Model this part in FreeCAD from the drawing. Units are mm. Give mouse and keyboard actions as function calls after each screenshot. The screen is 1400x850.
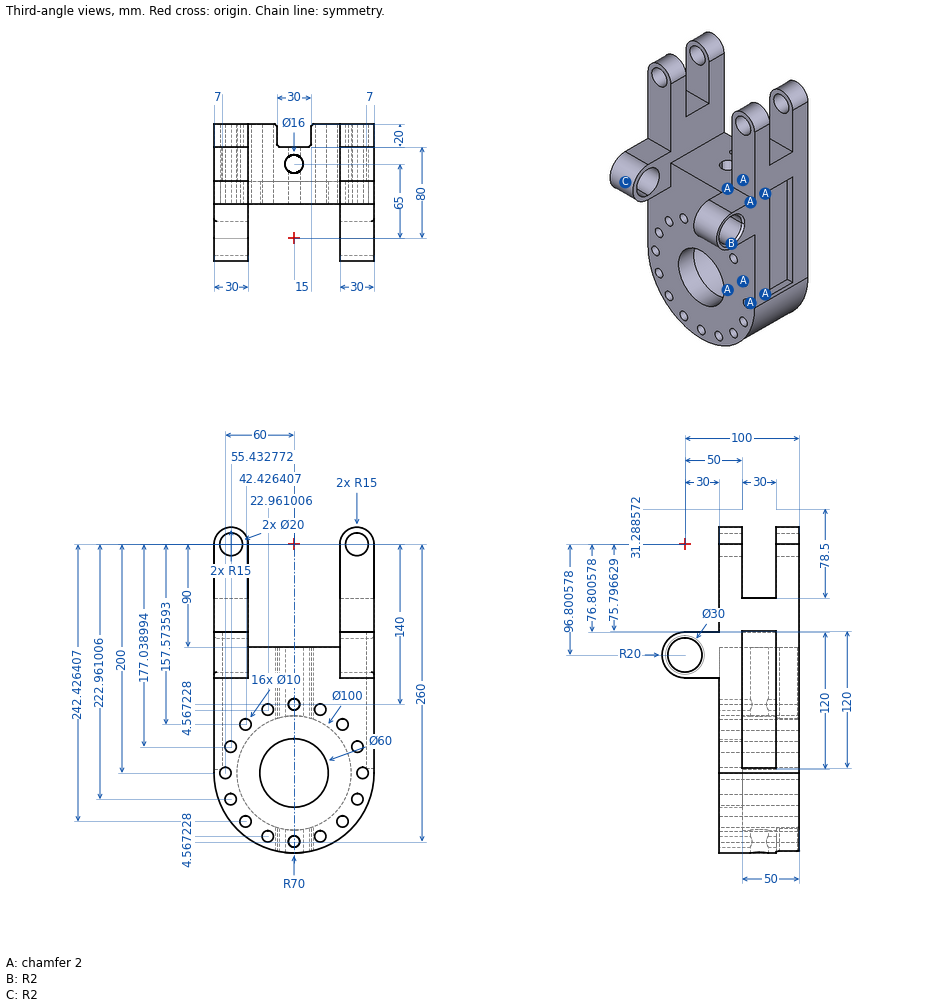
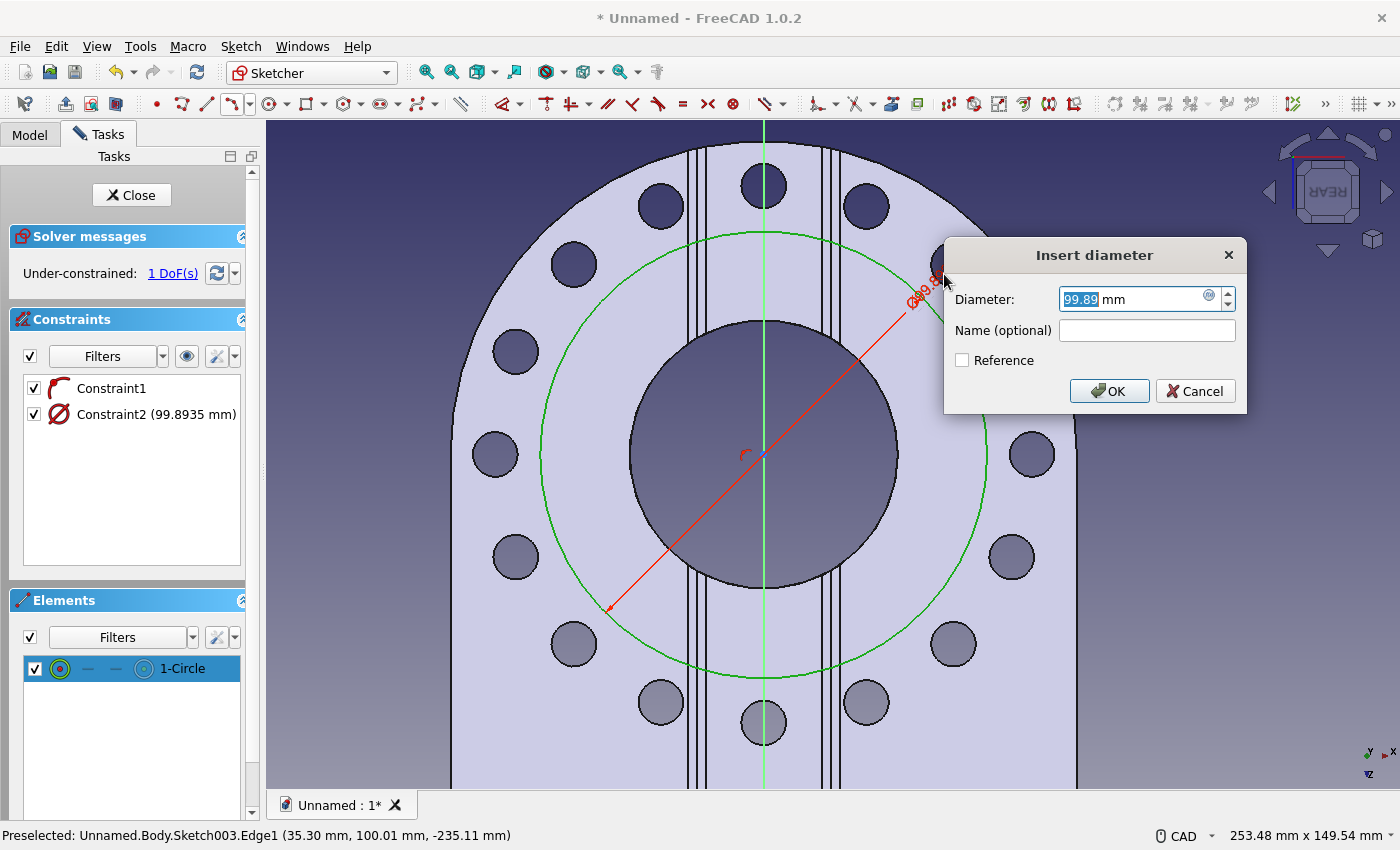
text(100)
key(Return)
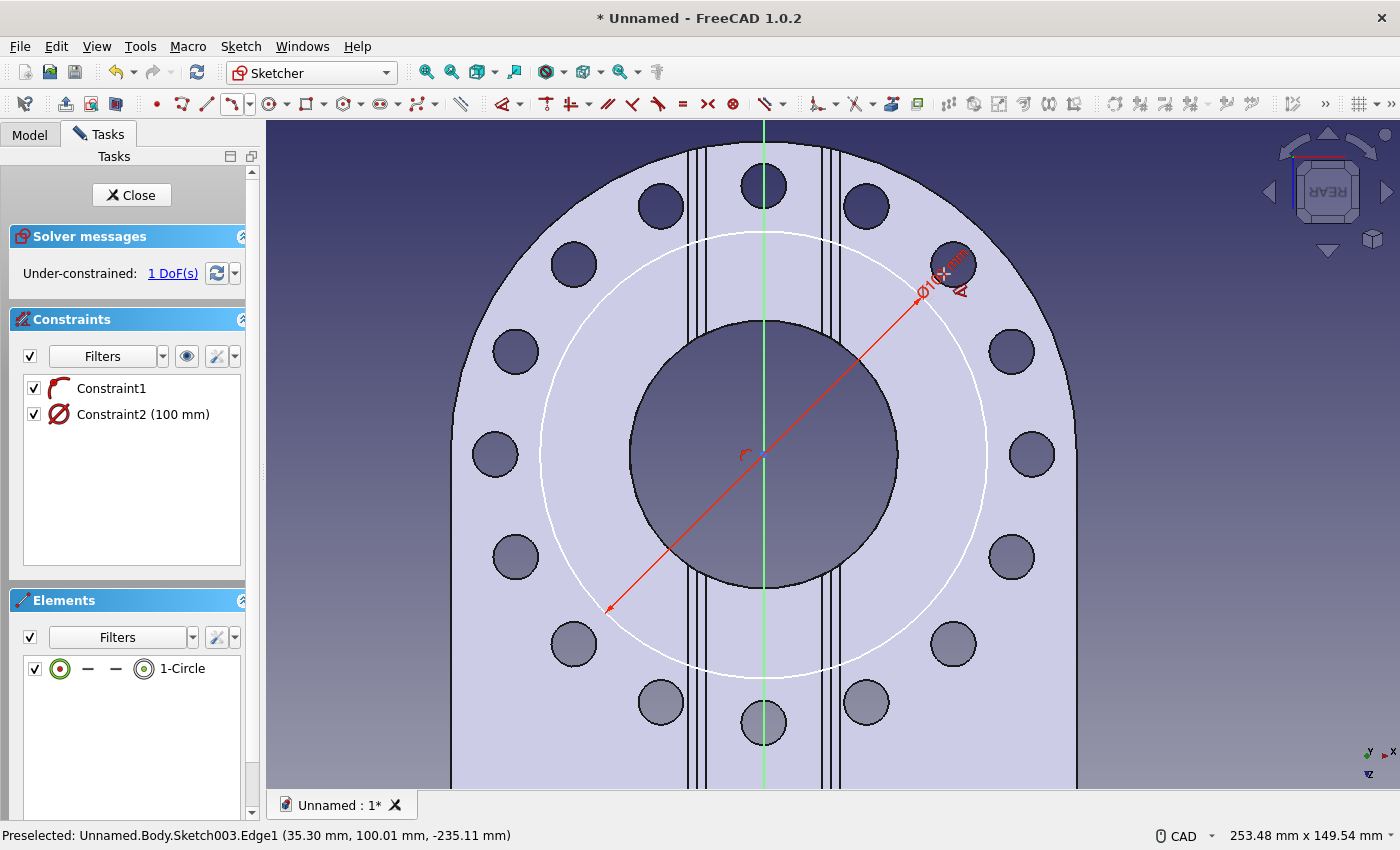
click(764, 455)
click(798, 608)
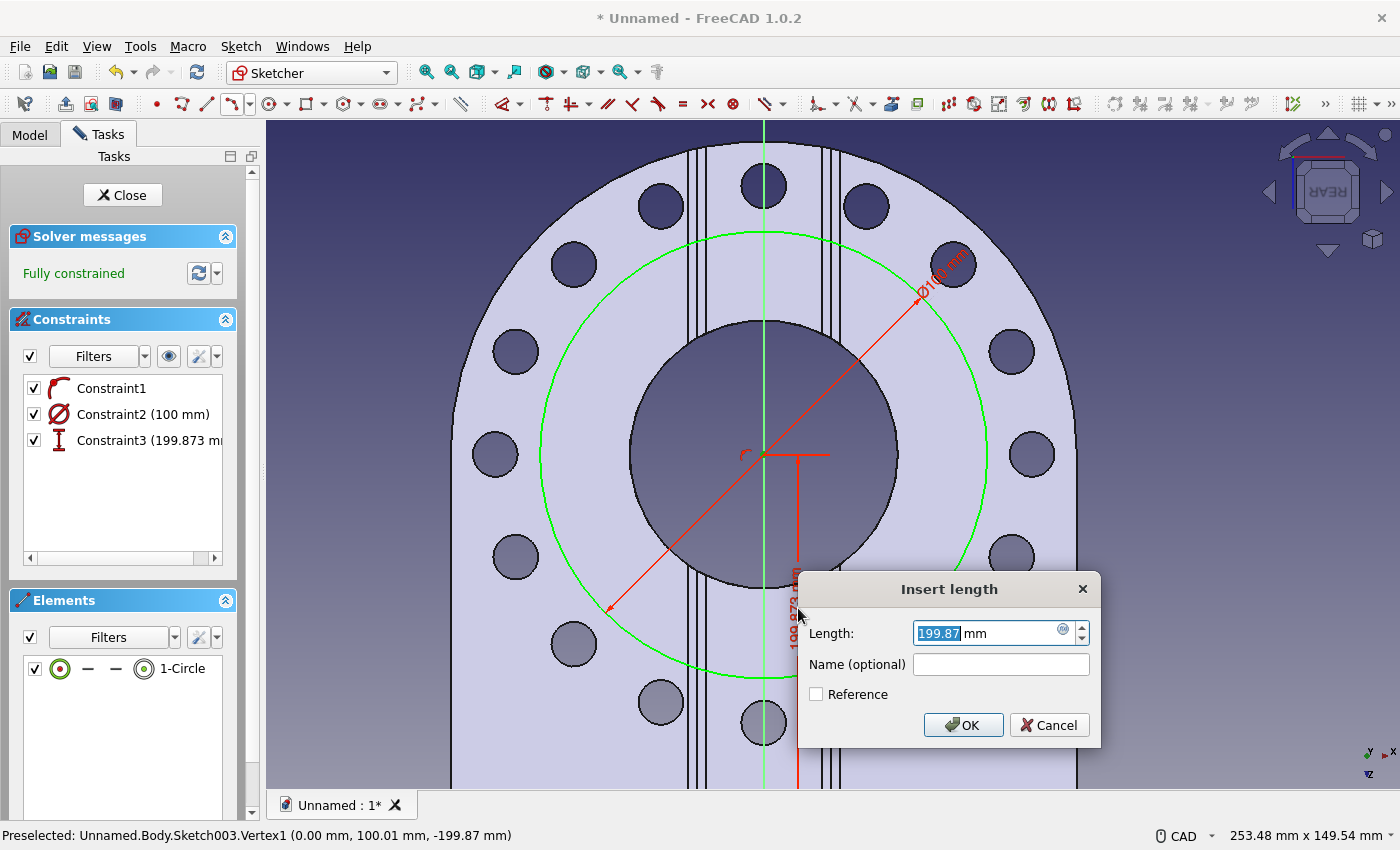
text(200)
key(Return)
key(Escape)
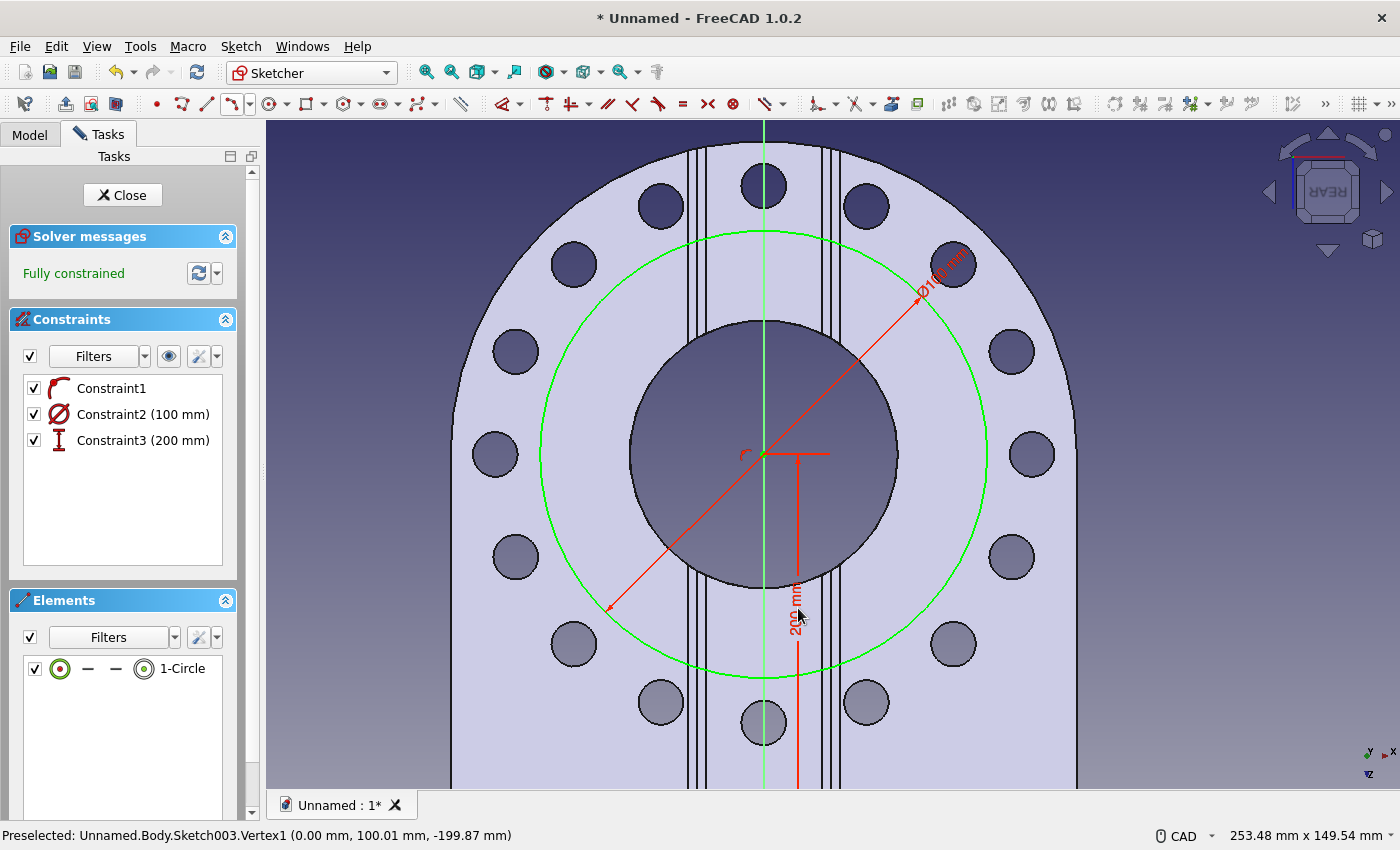
click(123, 195)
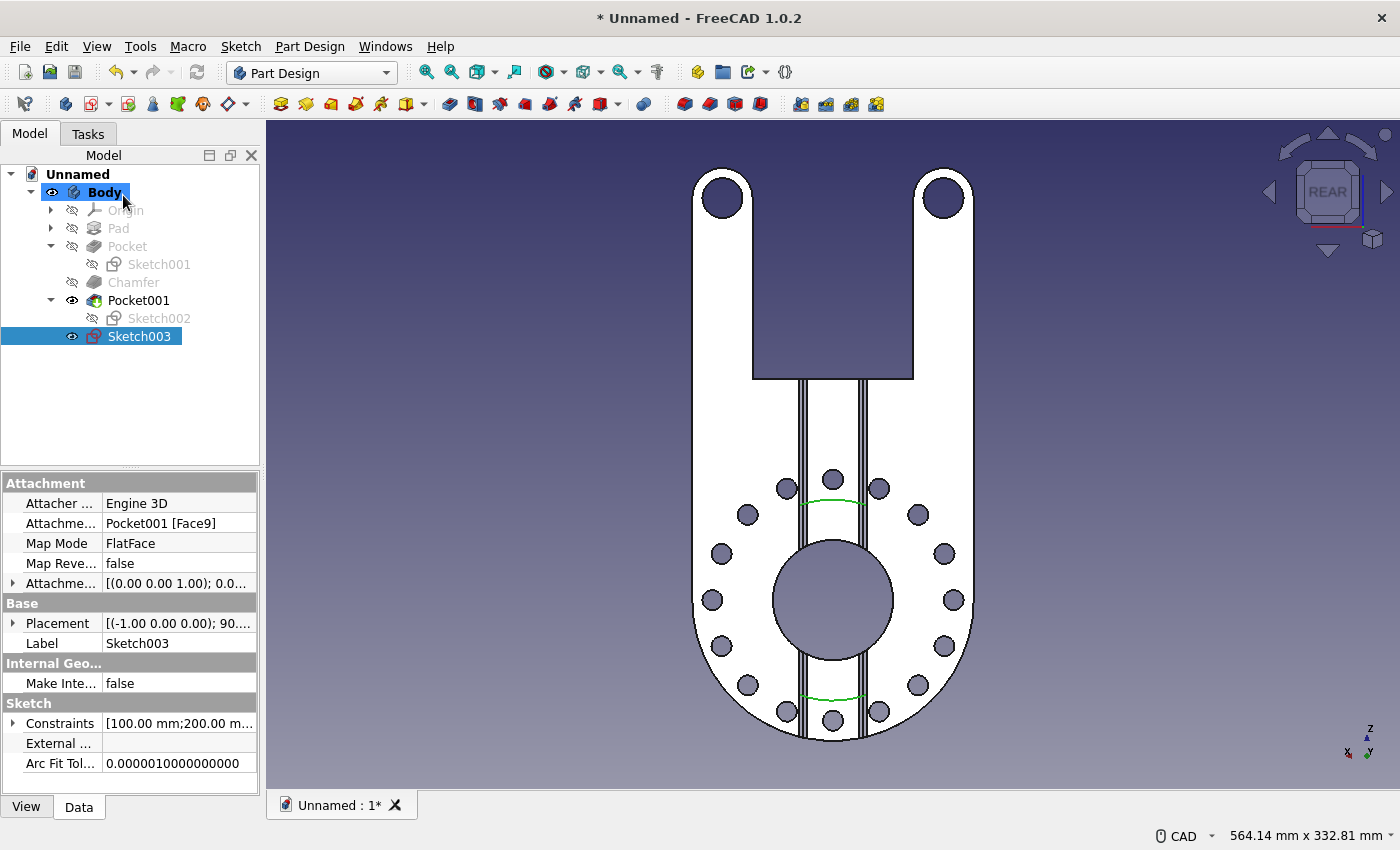
click(450, 104)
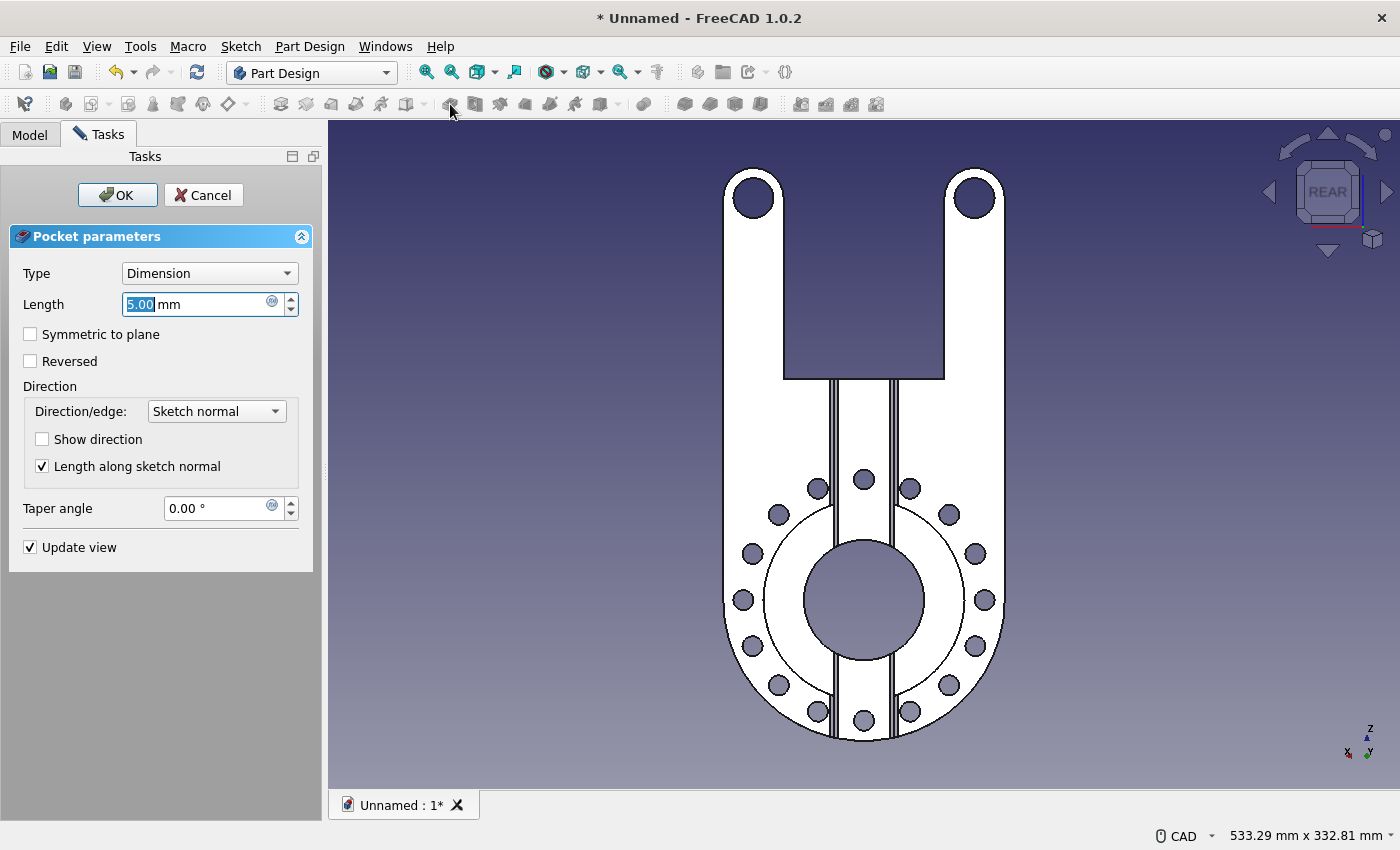
text(50)
key(Tab)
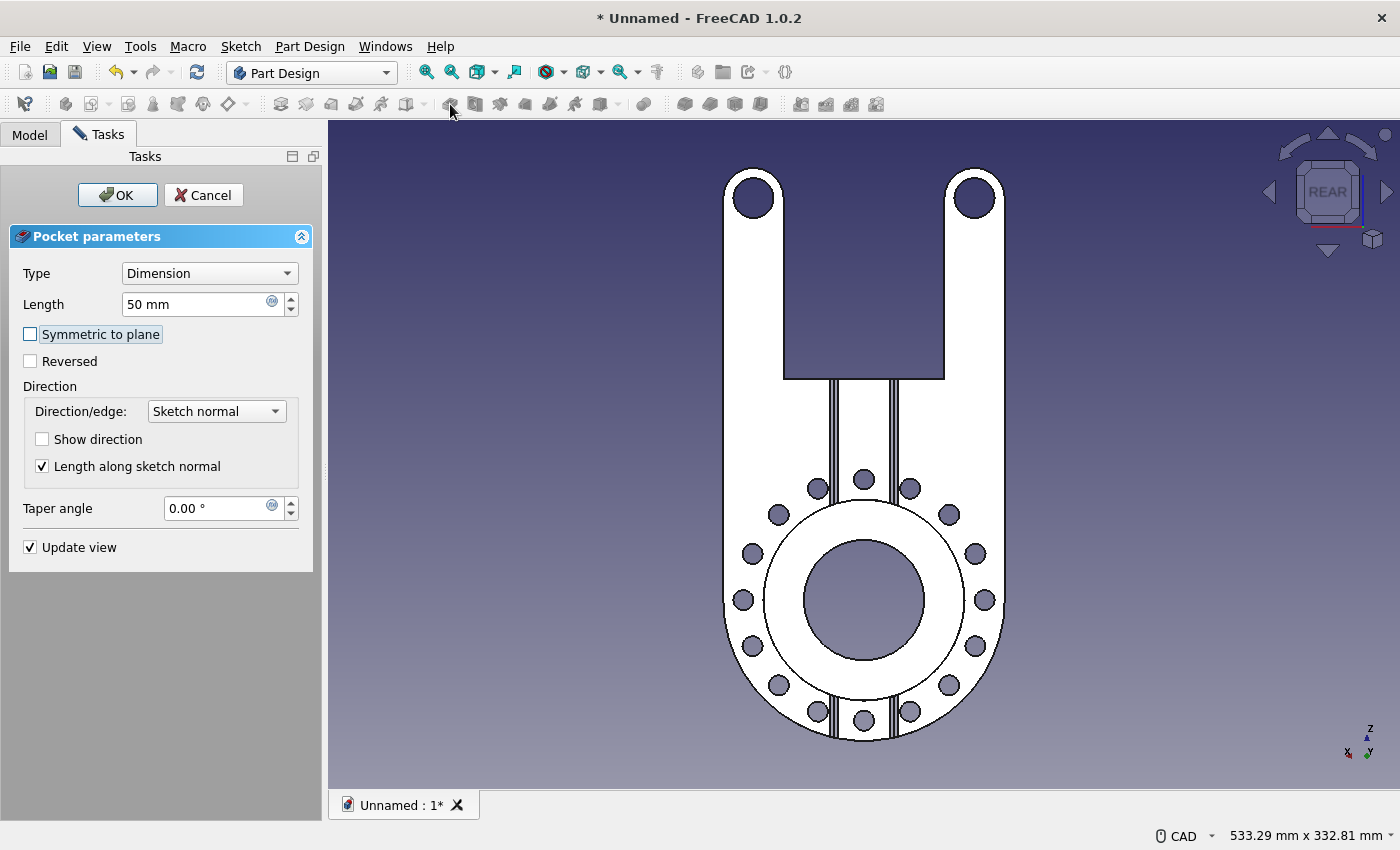
click(118, 195)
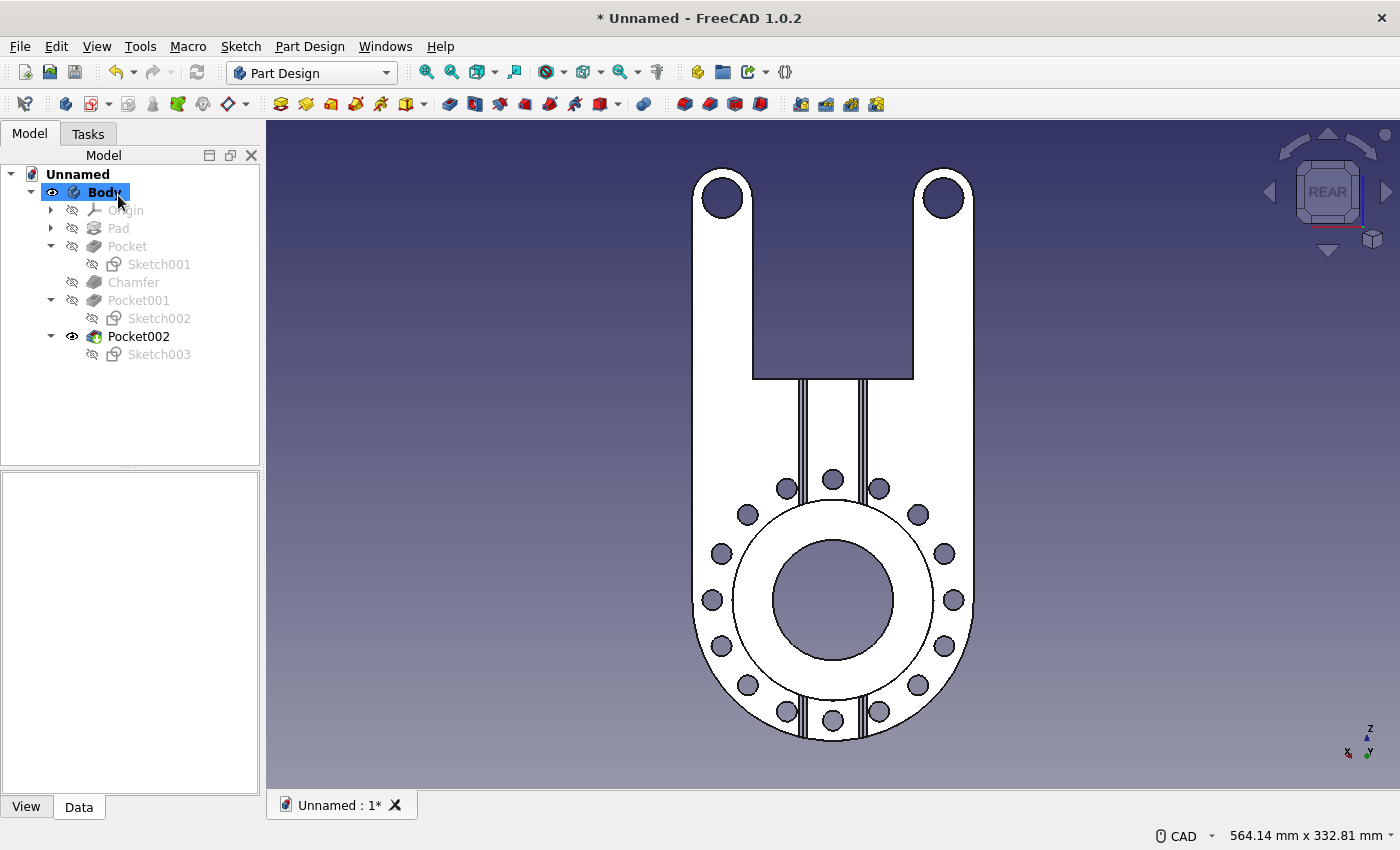
key(6)